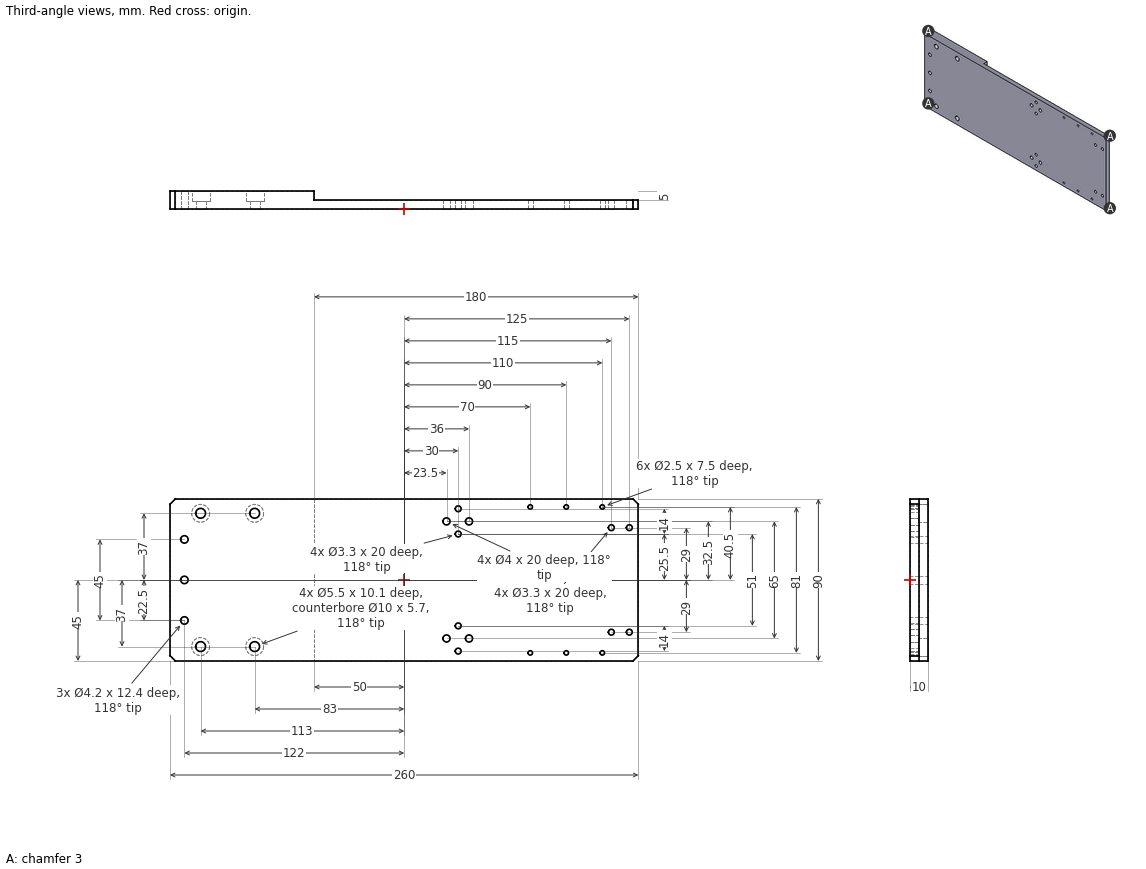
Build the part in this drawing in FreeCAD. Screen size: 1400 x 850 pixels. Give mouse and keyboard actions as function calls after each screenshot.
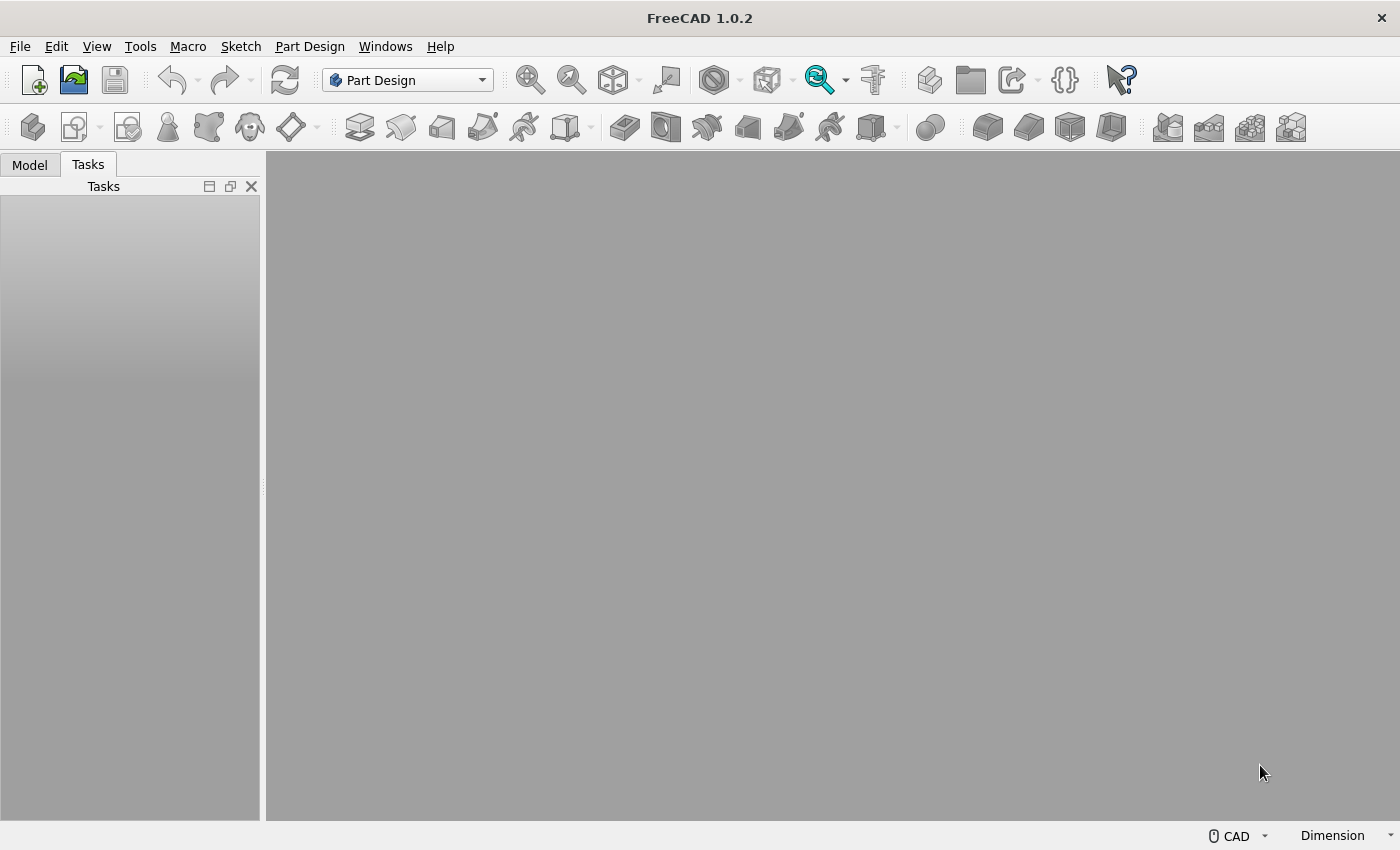
click(33, 80)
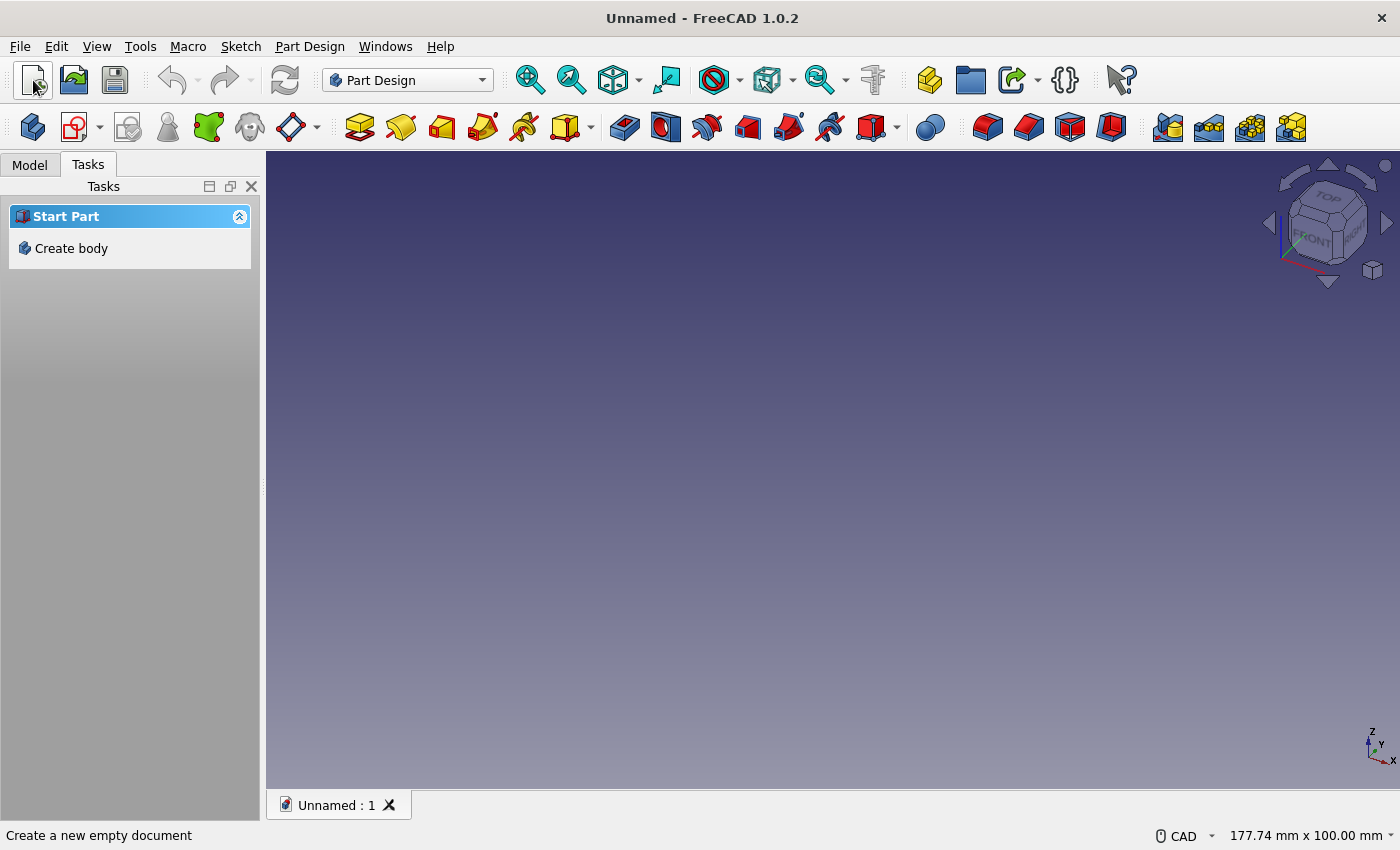
click(74, 128)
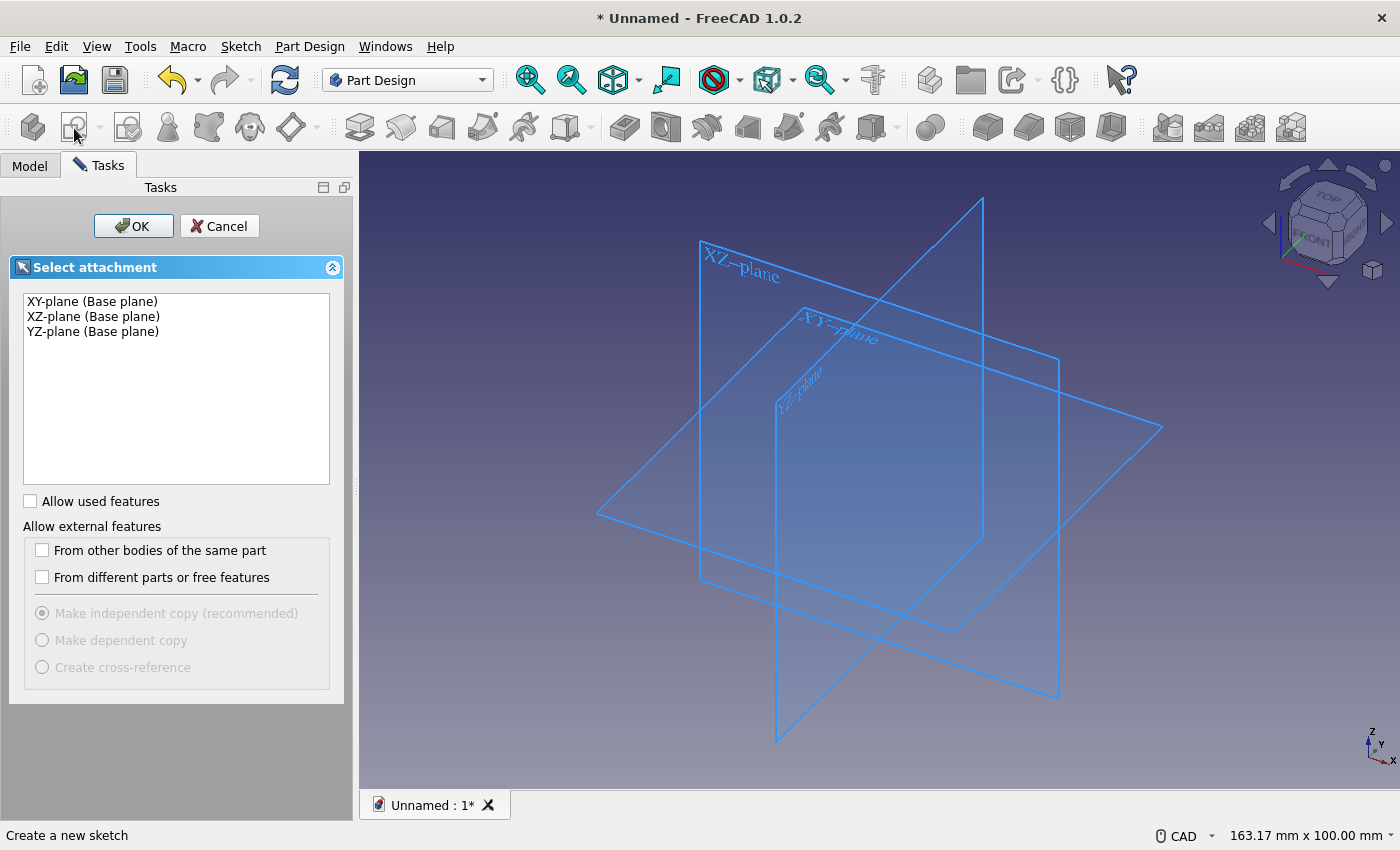
click(84, 316)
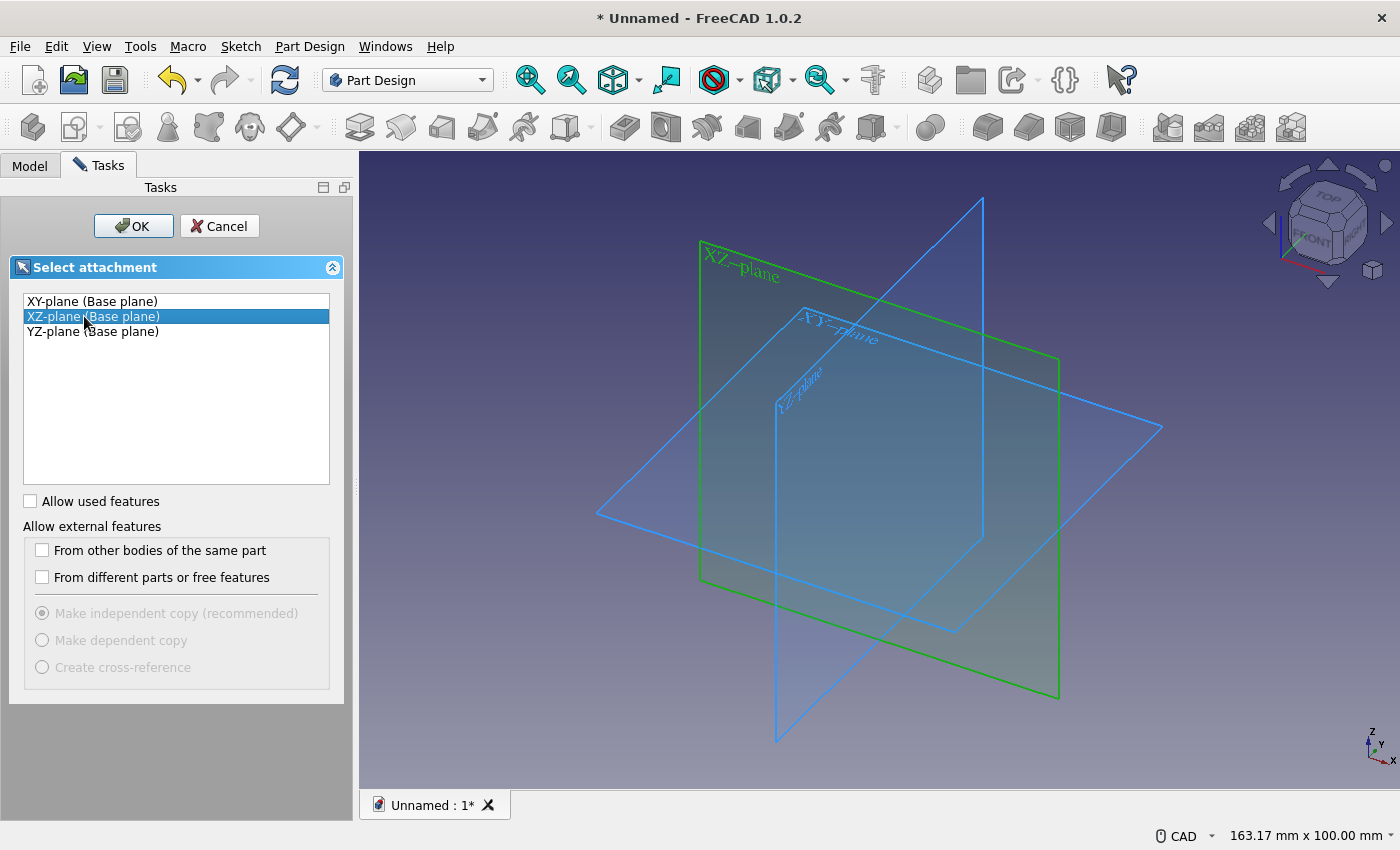
click(134, 226)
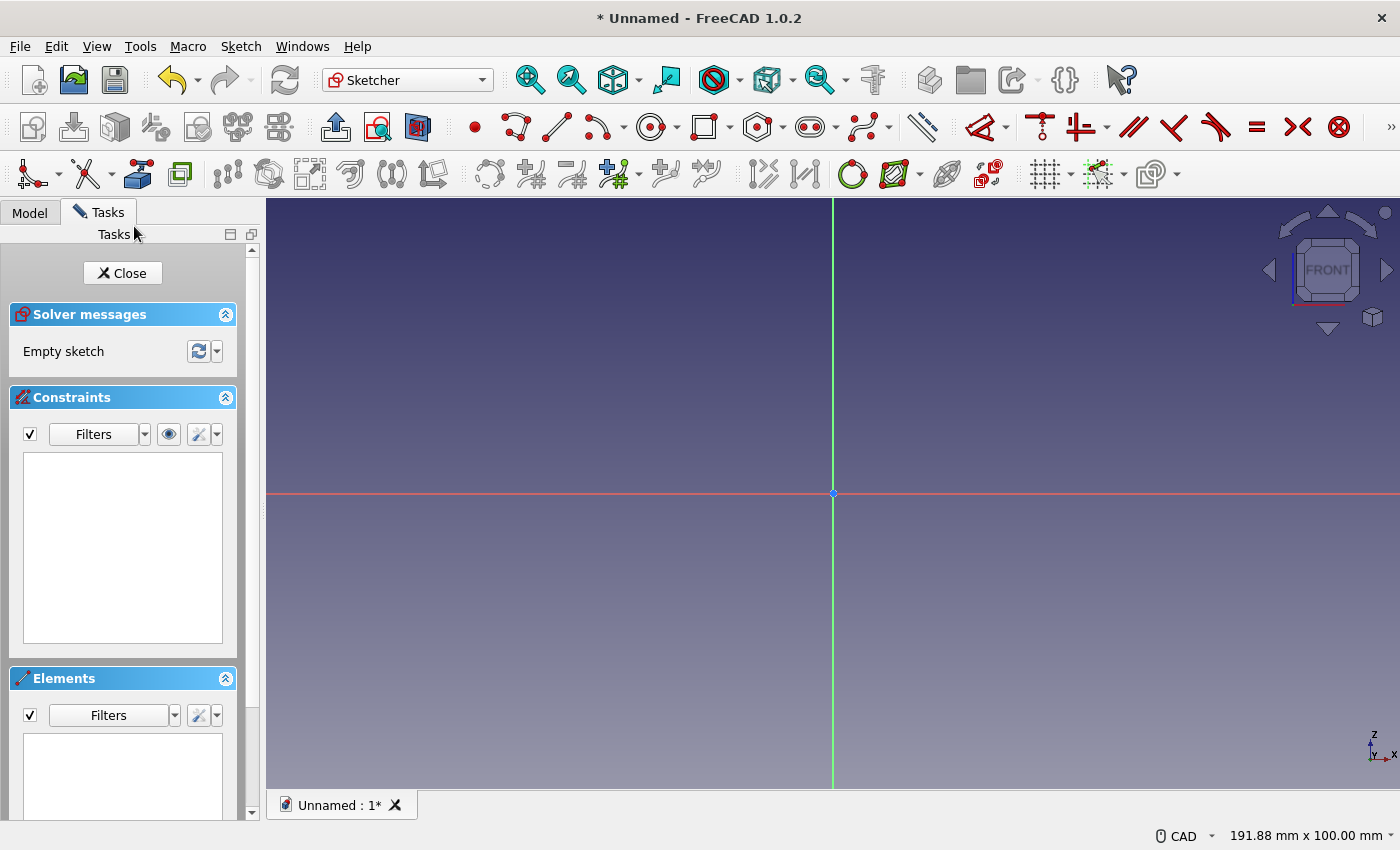
scroll(709, 494, down, 4)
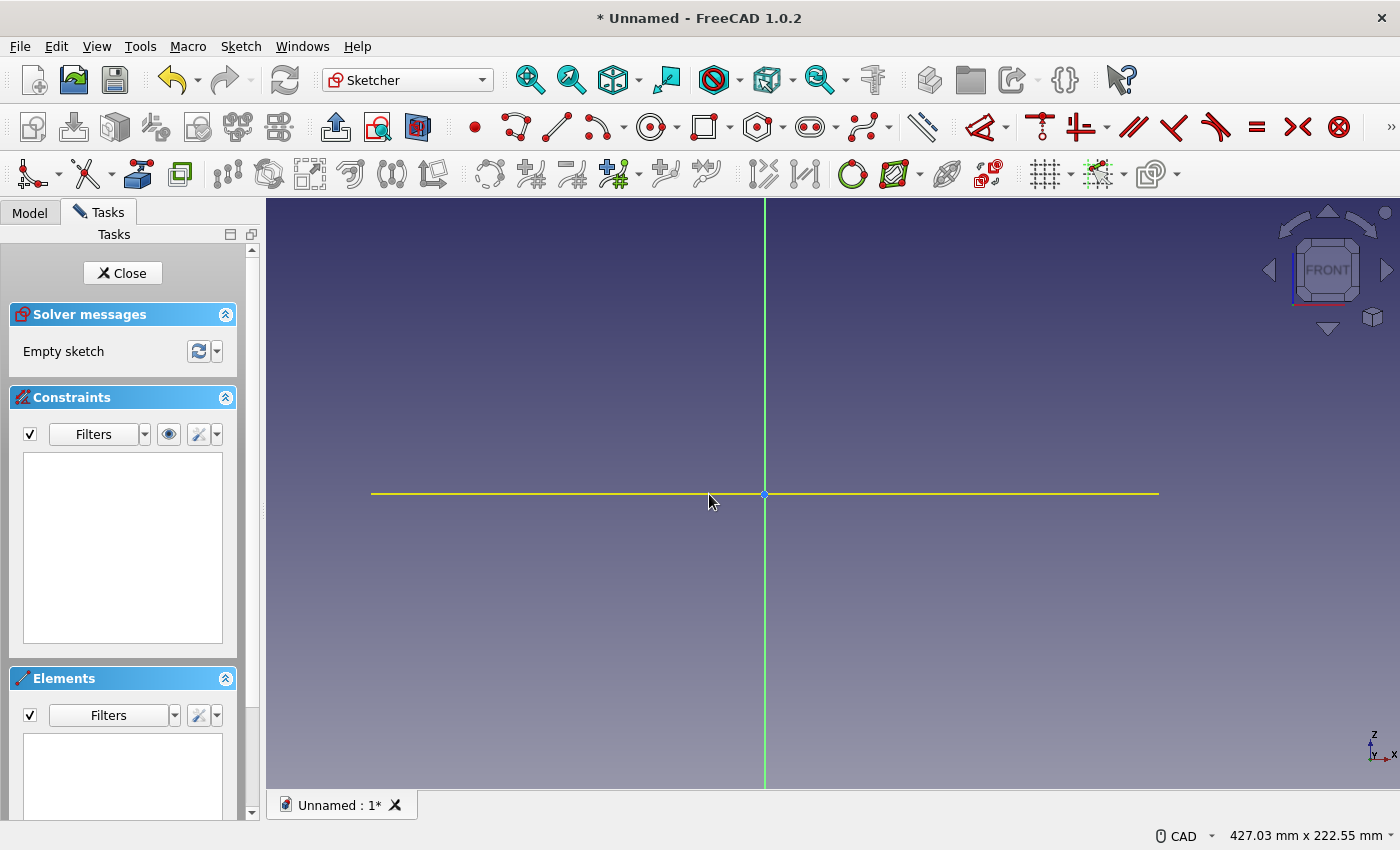
key(g)
key(v)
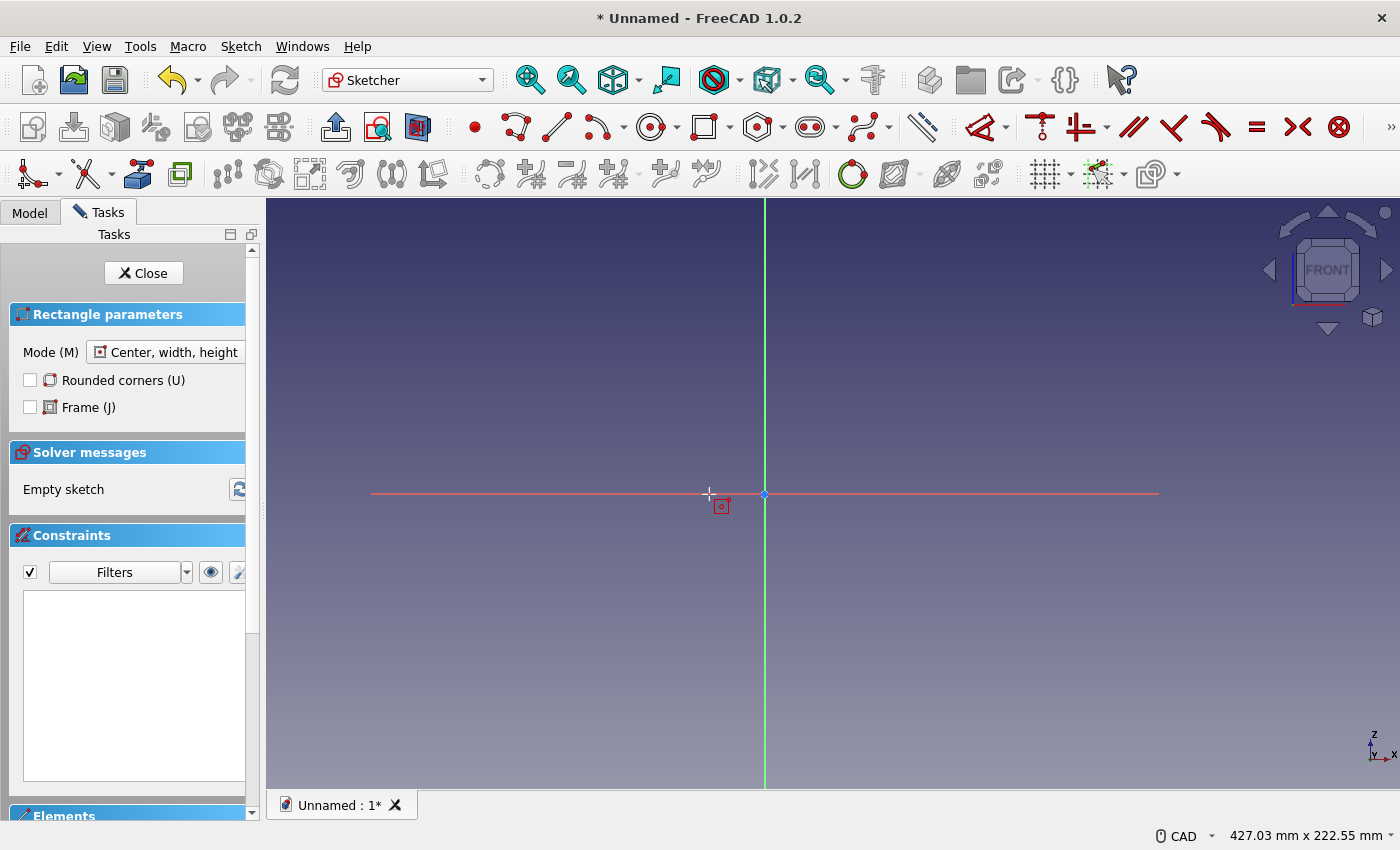
click(765, 494)
click(1110, 375)
key(Escape)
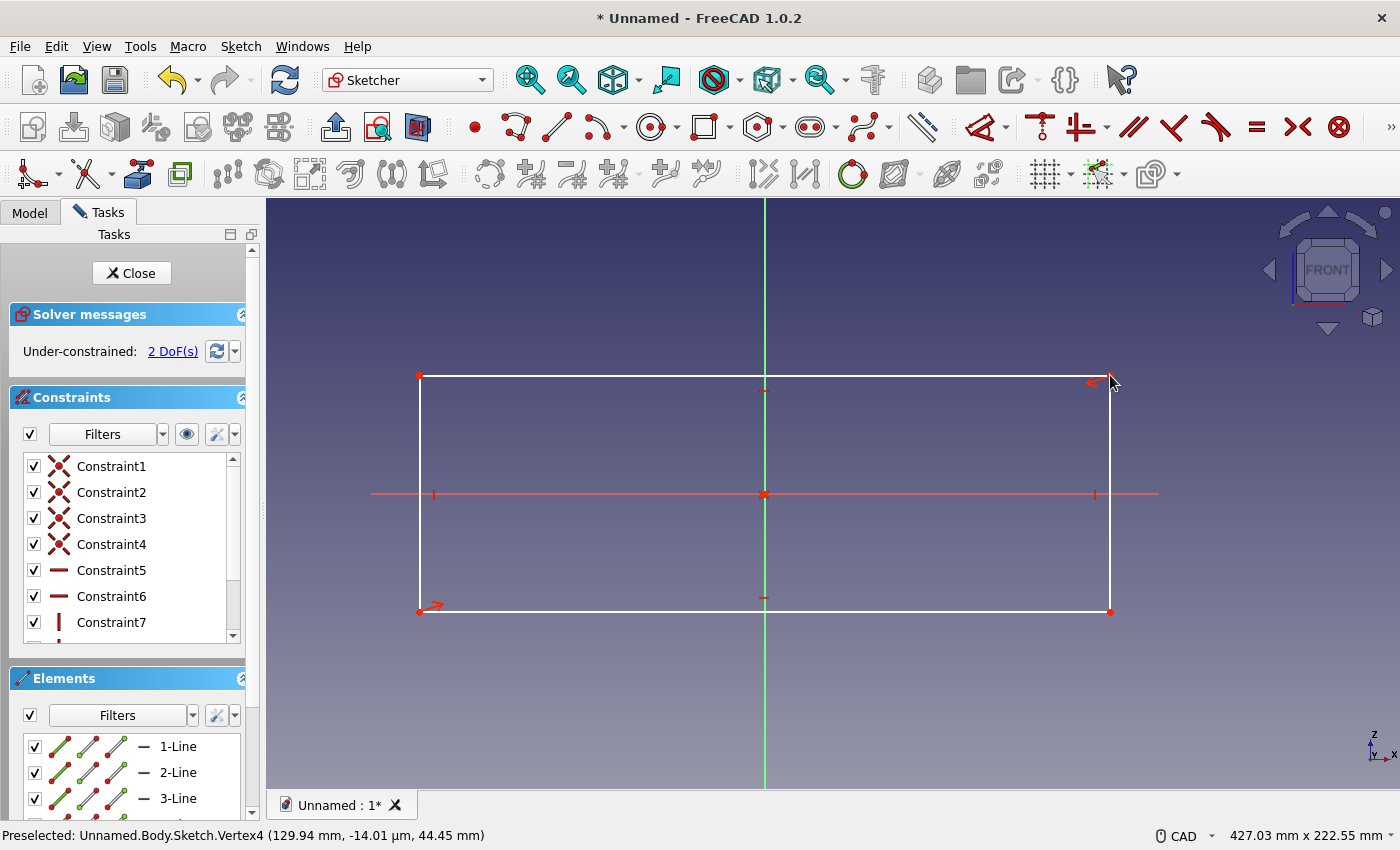
click(980, 128)